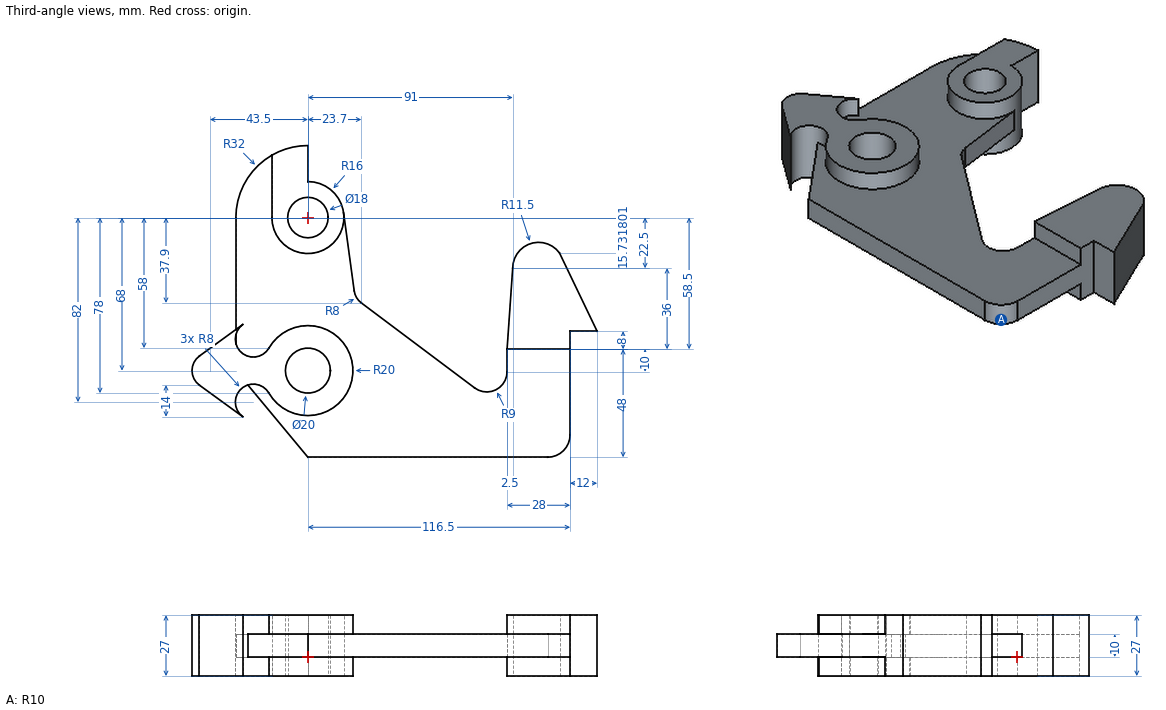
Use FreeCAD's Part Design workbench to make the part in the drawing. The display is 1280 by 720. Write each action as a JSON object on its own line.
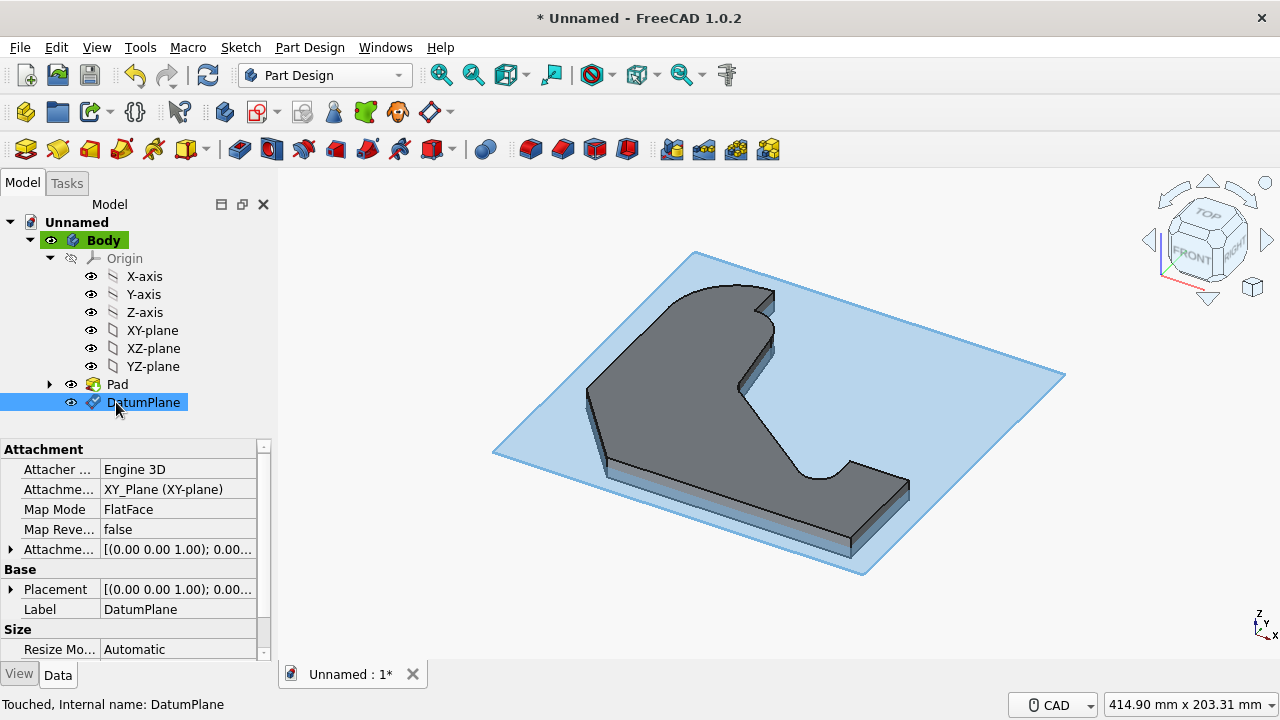
{"action": "left_click", "coordinate": [258, 112]}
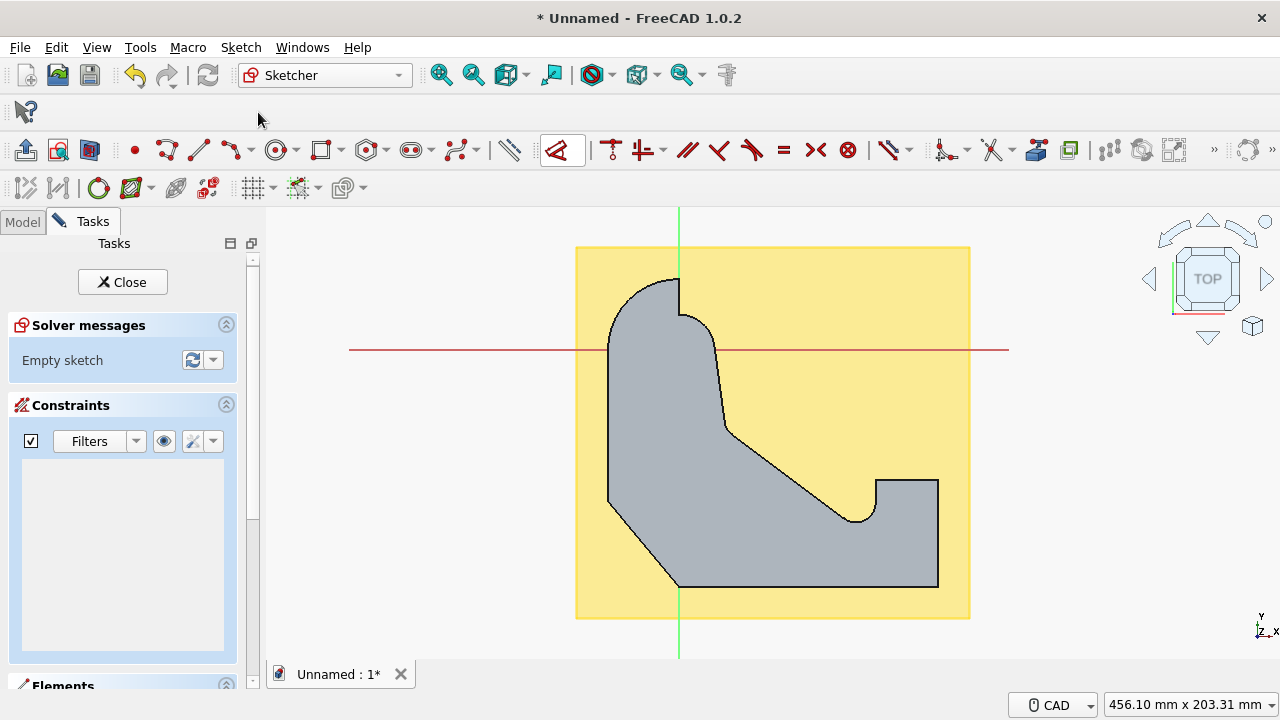
{"action": "key", "text": "q s"}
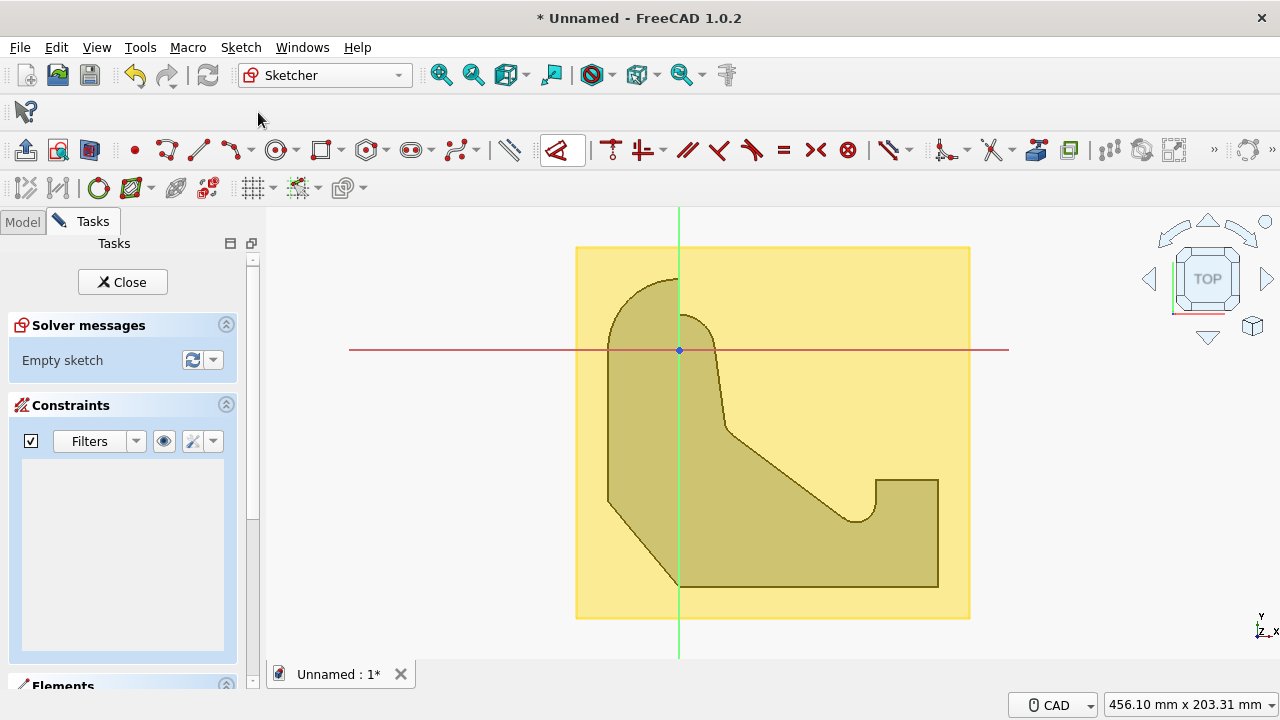
{"action": "scroll", "coordinate": [656, 266], "scroll_direction": "up", "scroll_amount": 5}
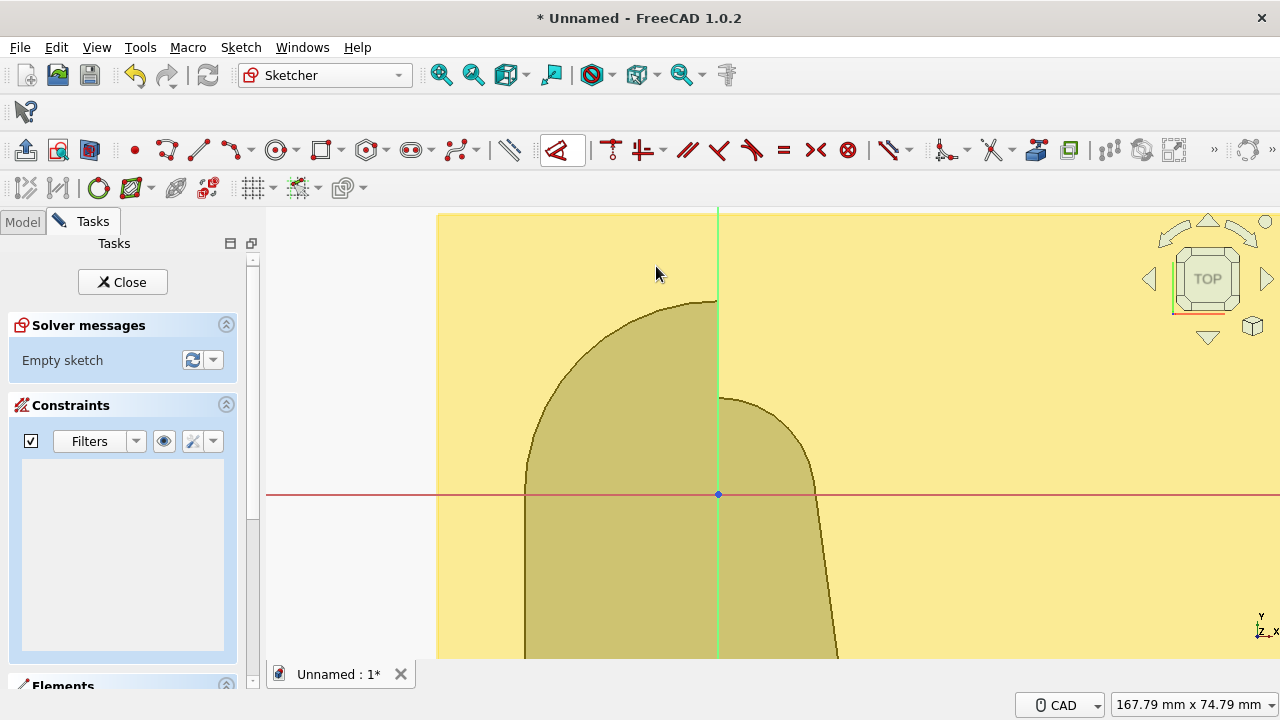
{"action": "key", "text": "g l"}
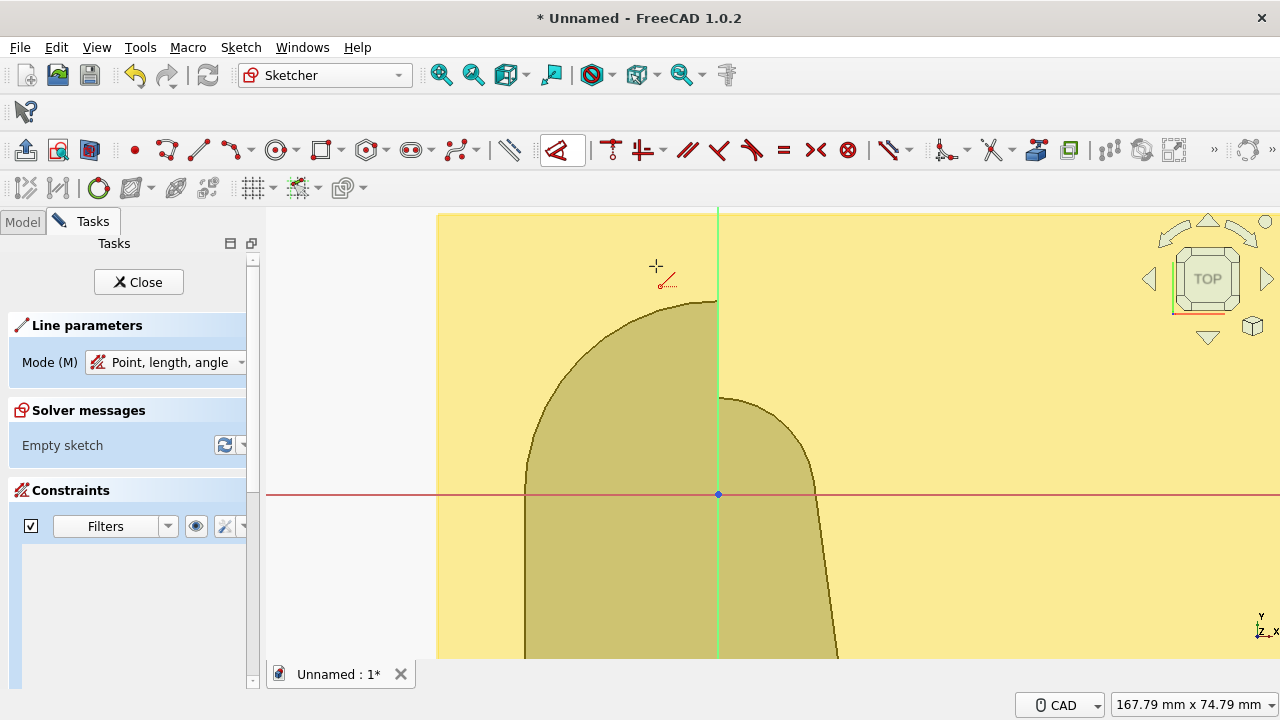
{"action": "left_click", "coordinate": [718, 398]}
{"action": "left_click", "coordinate": [709, 301]}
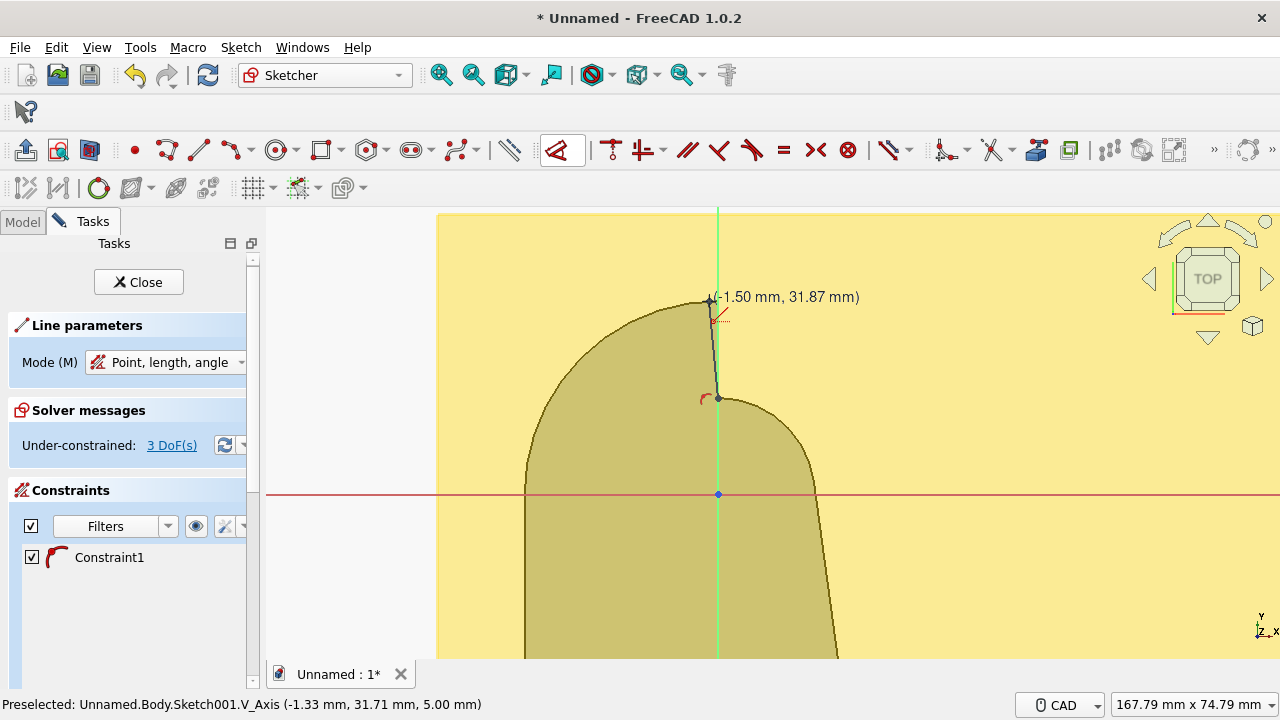
{"action": "left_click", "coordinate": [621, 327]}
{"action": "left_click", "coordinate": [621, 495]}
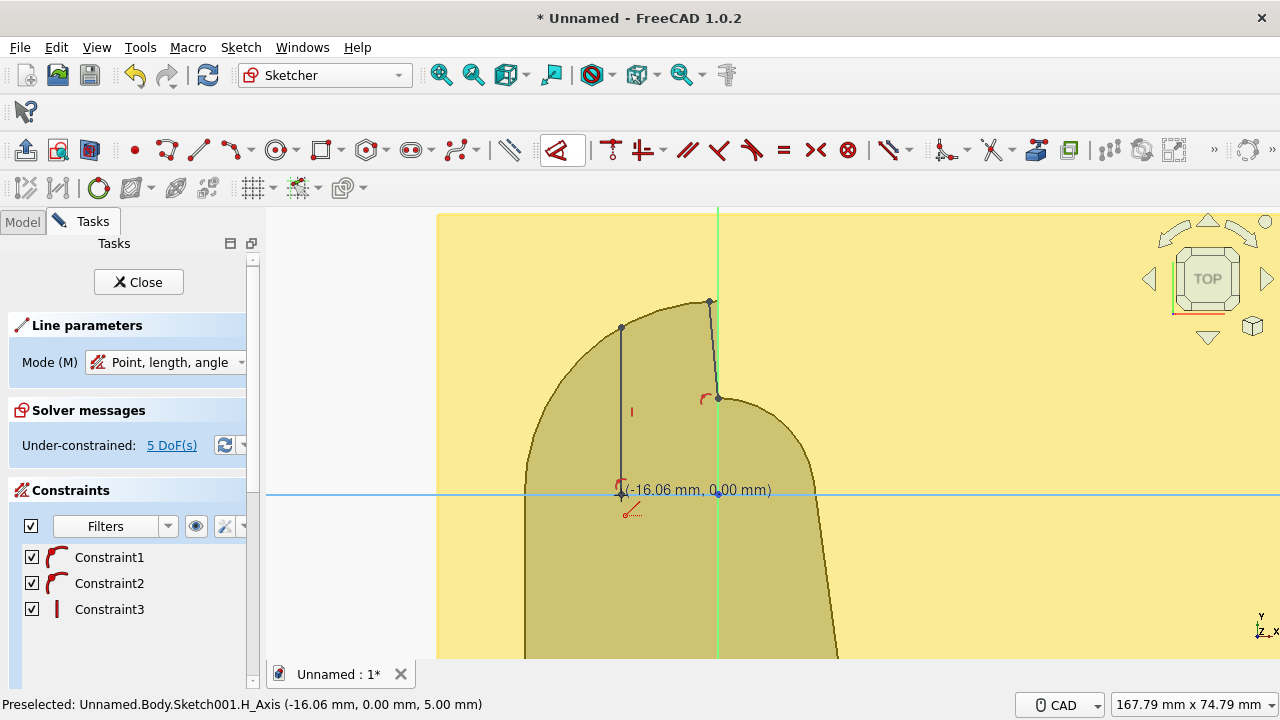
{"action": "left_click", "coordinate": [232, 150]}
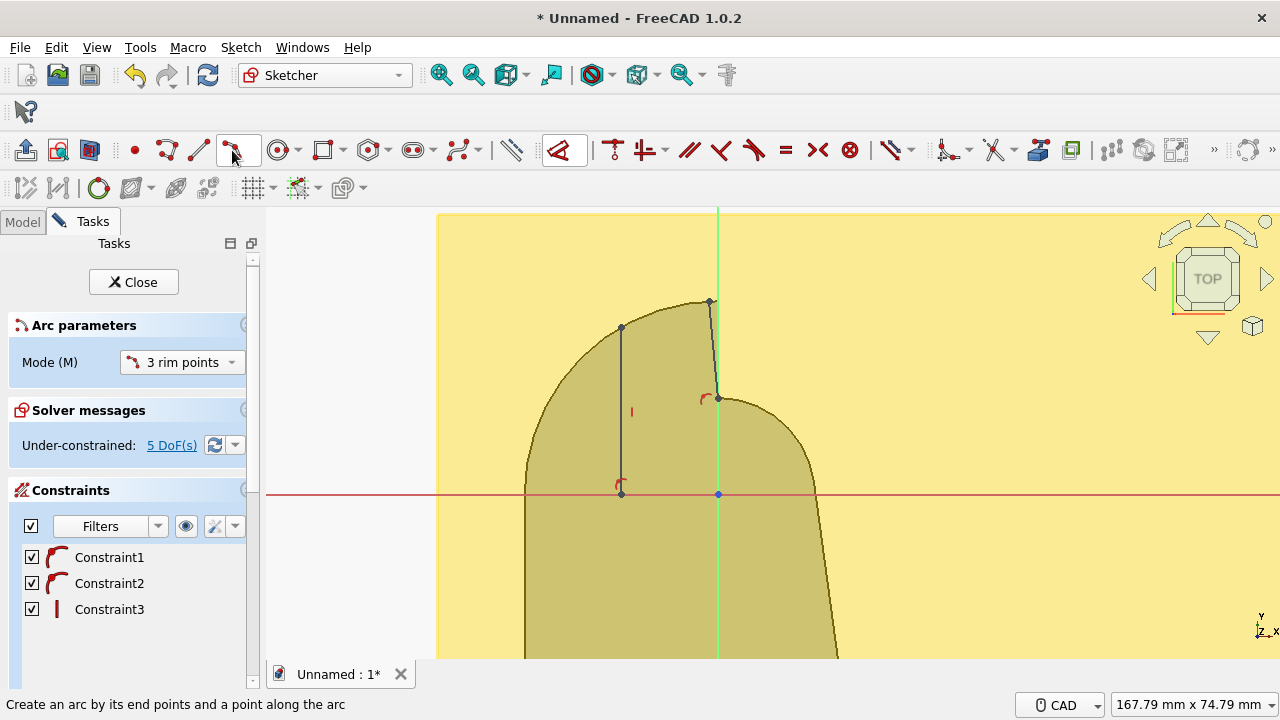
{"action": "left_click", "coordinate": [709, 302]}
{"action": "left_click", "coordinate": [621, 328]}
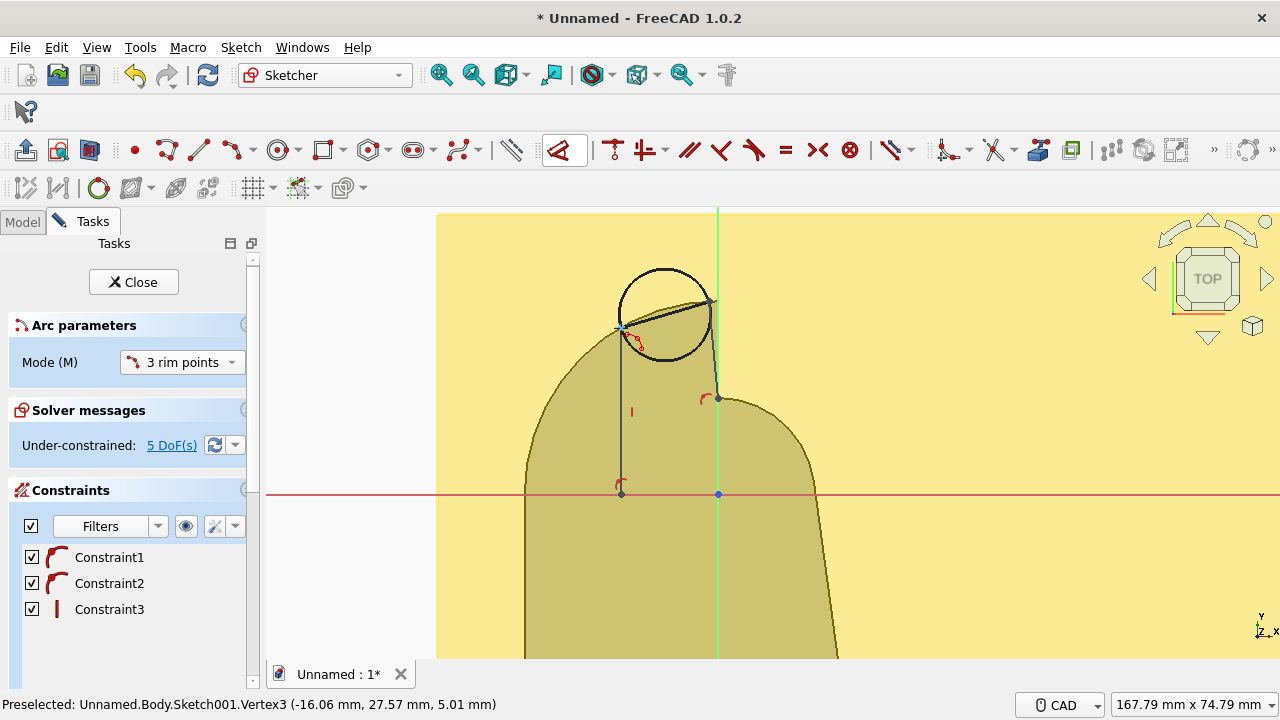
{"action": "scroll", "coordinate": [668, 308], "scroll_direction": "up", "scroll_amount": 5}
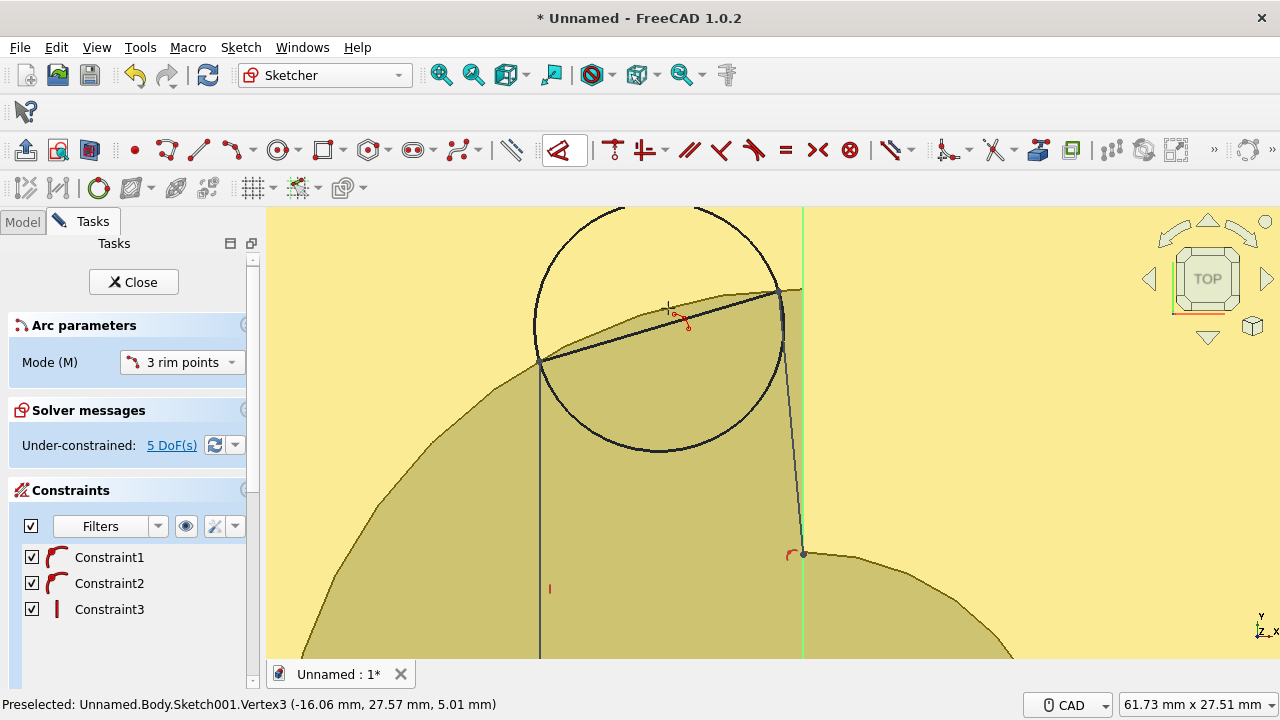
{"action": "left_click", "coordinate": [667, 307]}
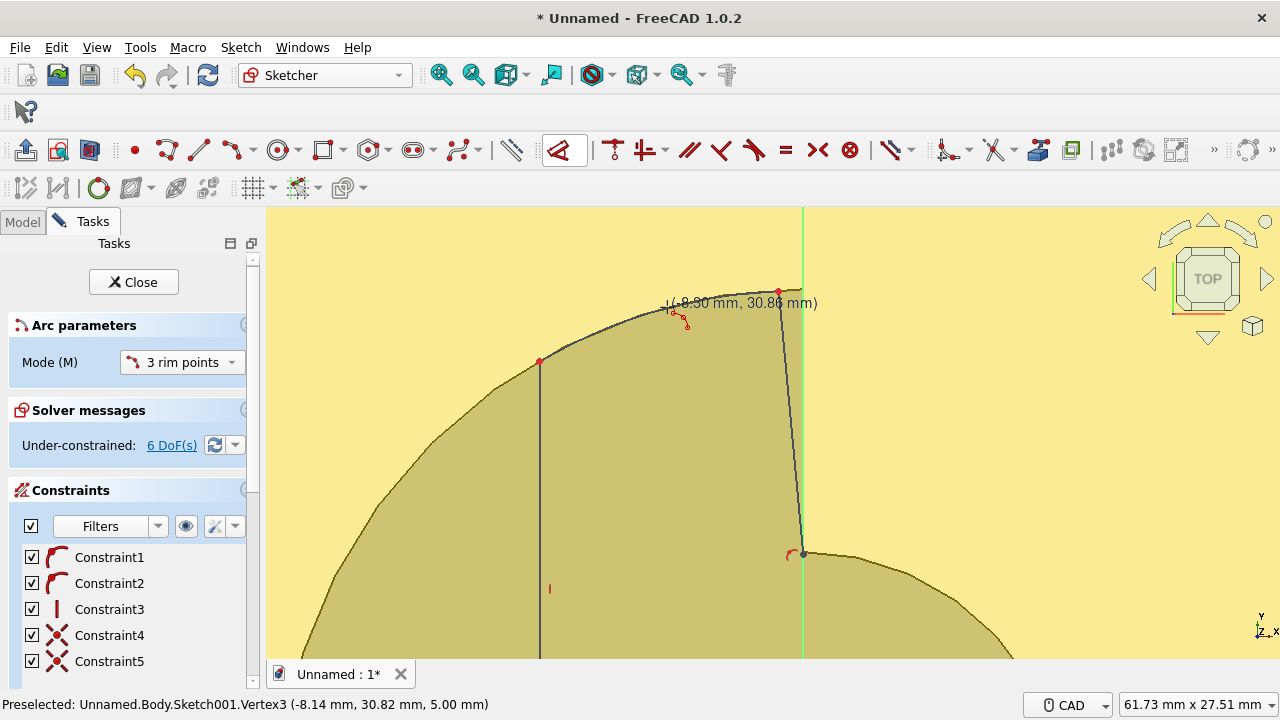
{"action": "scroll", "coordinate": [669, 310], "scroll_direction": "down", "scroll_amount": 5}